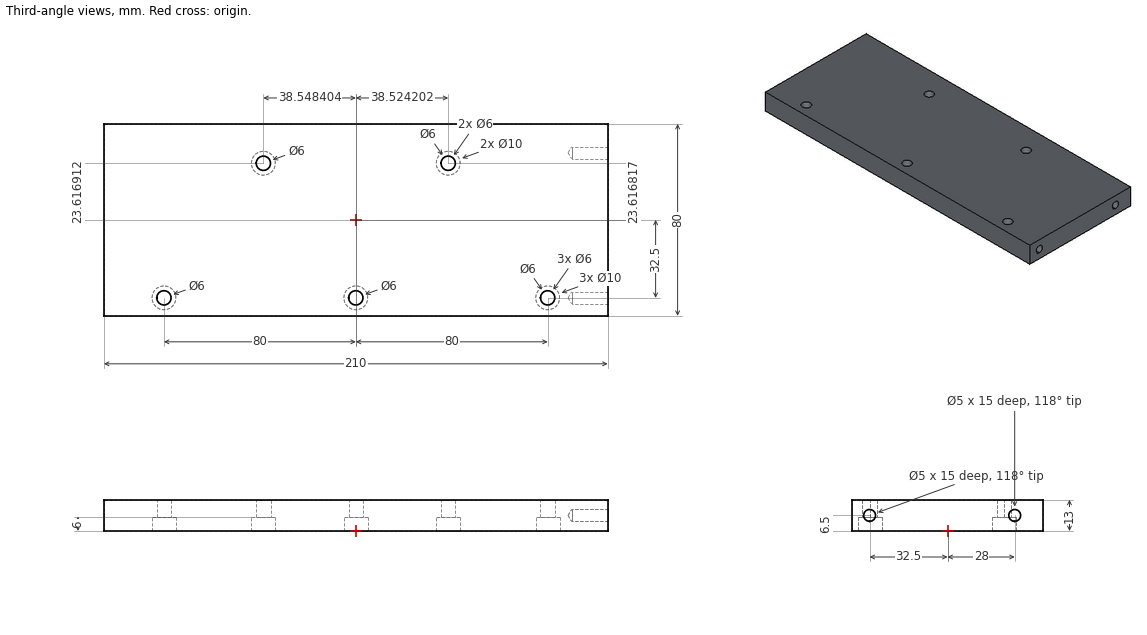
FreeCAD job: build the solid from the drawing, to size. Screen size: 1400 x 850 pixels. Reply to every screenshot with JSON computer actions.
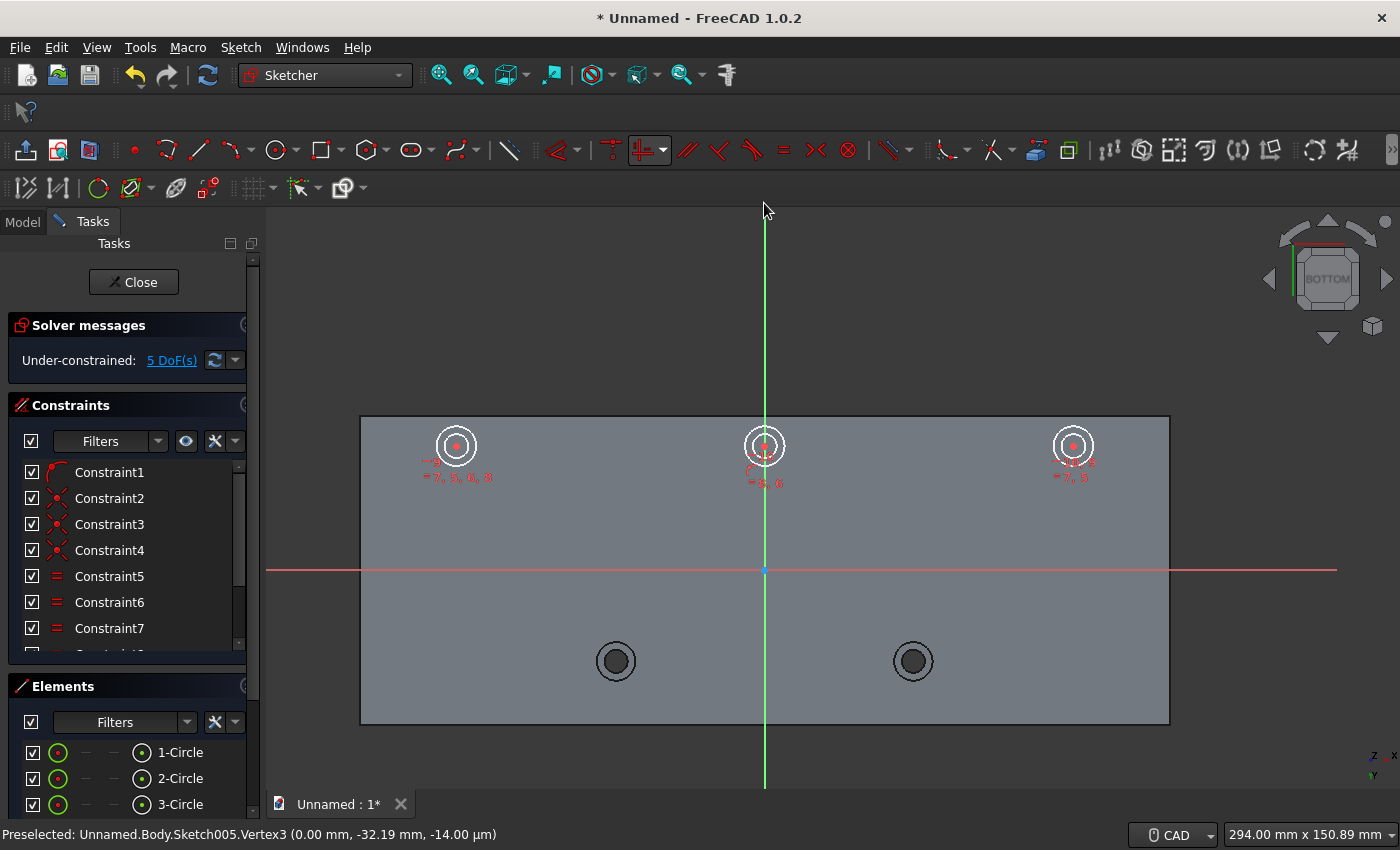
{"action": "key", "text": "d"}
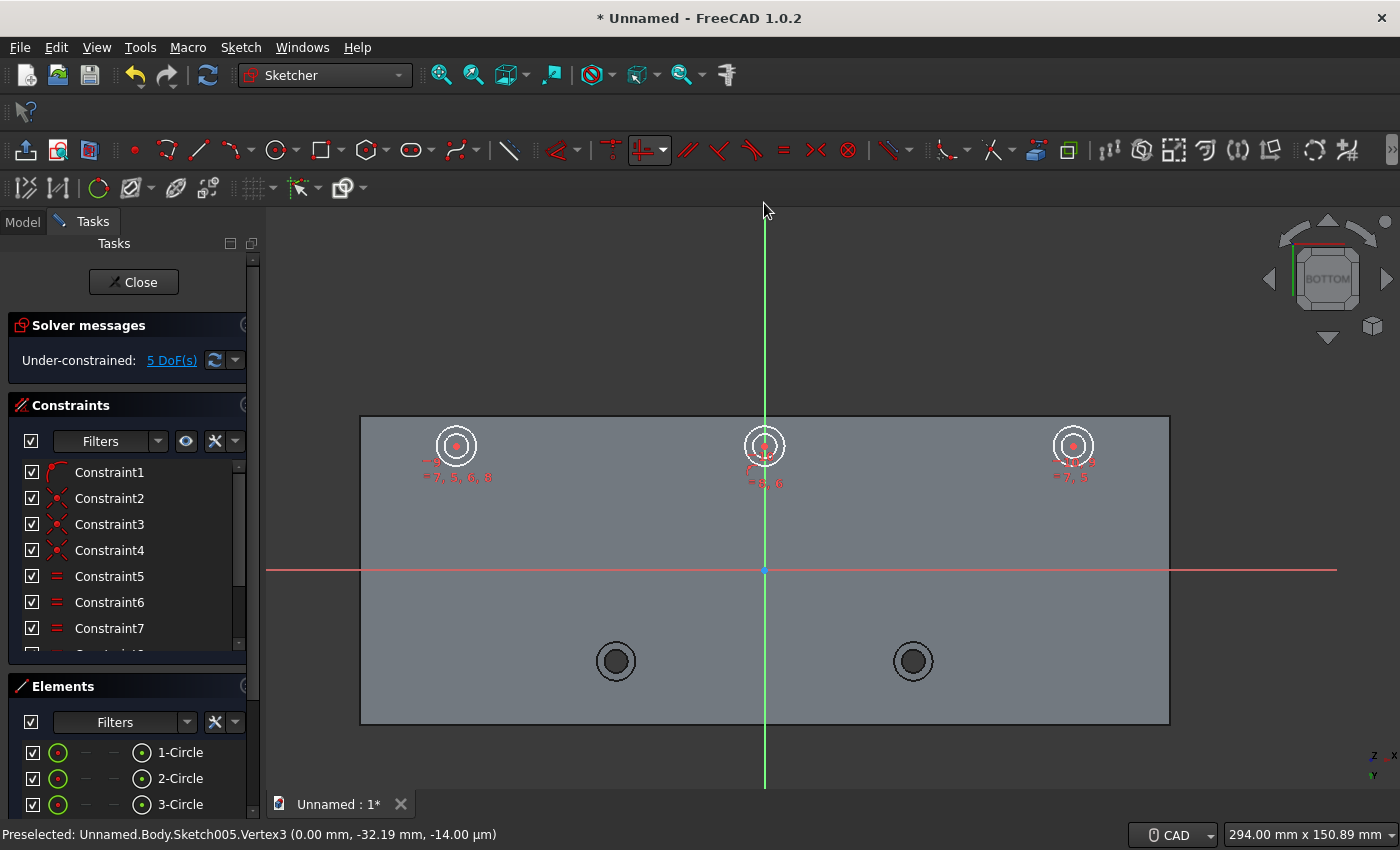
{"action": "scroll", "coordinate": [1059, 432], "scroll_direction": "up", "scroll_amount": 3}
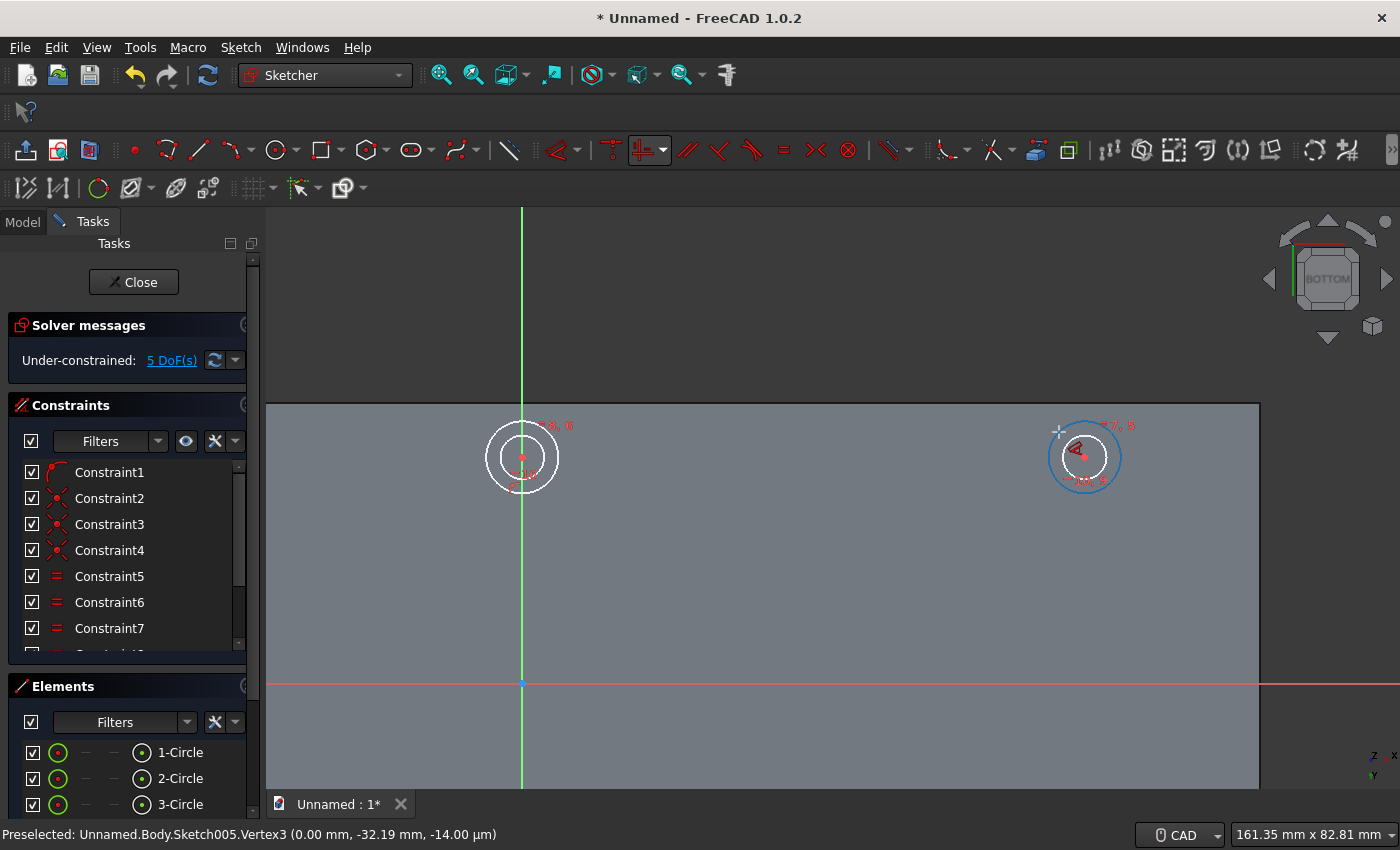
{"action": "left_click", "coordinate": [1059, 432]}
{"action": "left_click", "coordinate": [1036, 410]}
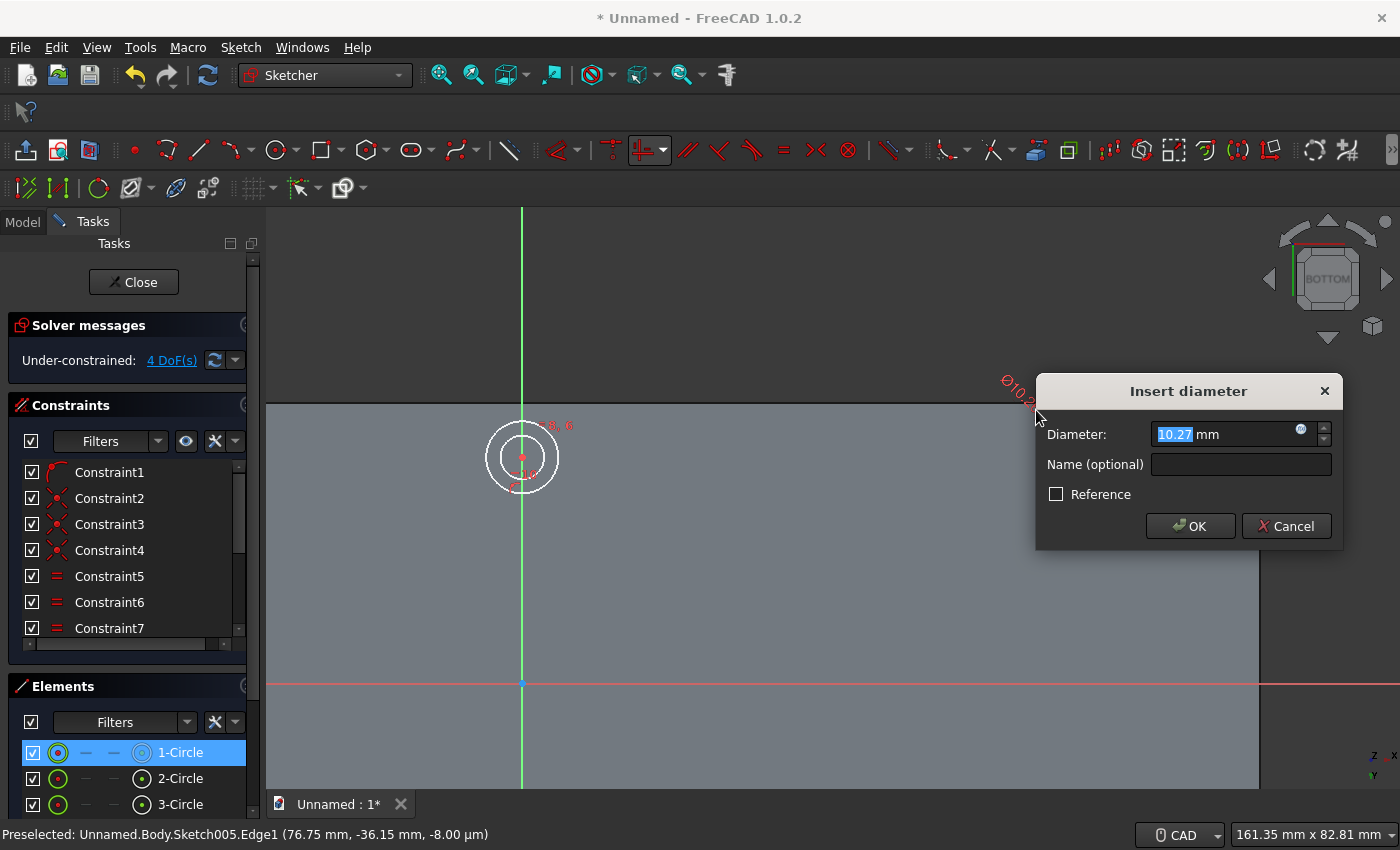
{"action": "type", "text": "10"}
{"action": "key", "text": "Return"}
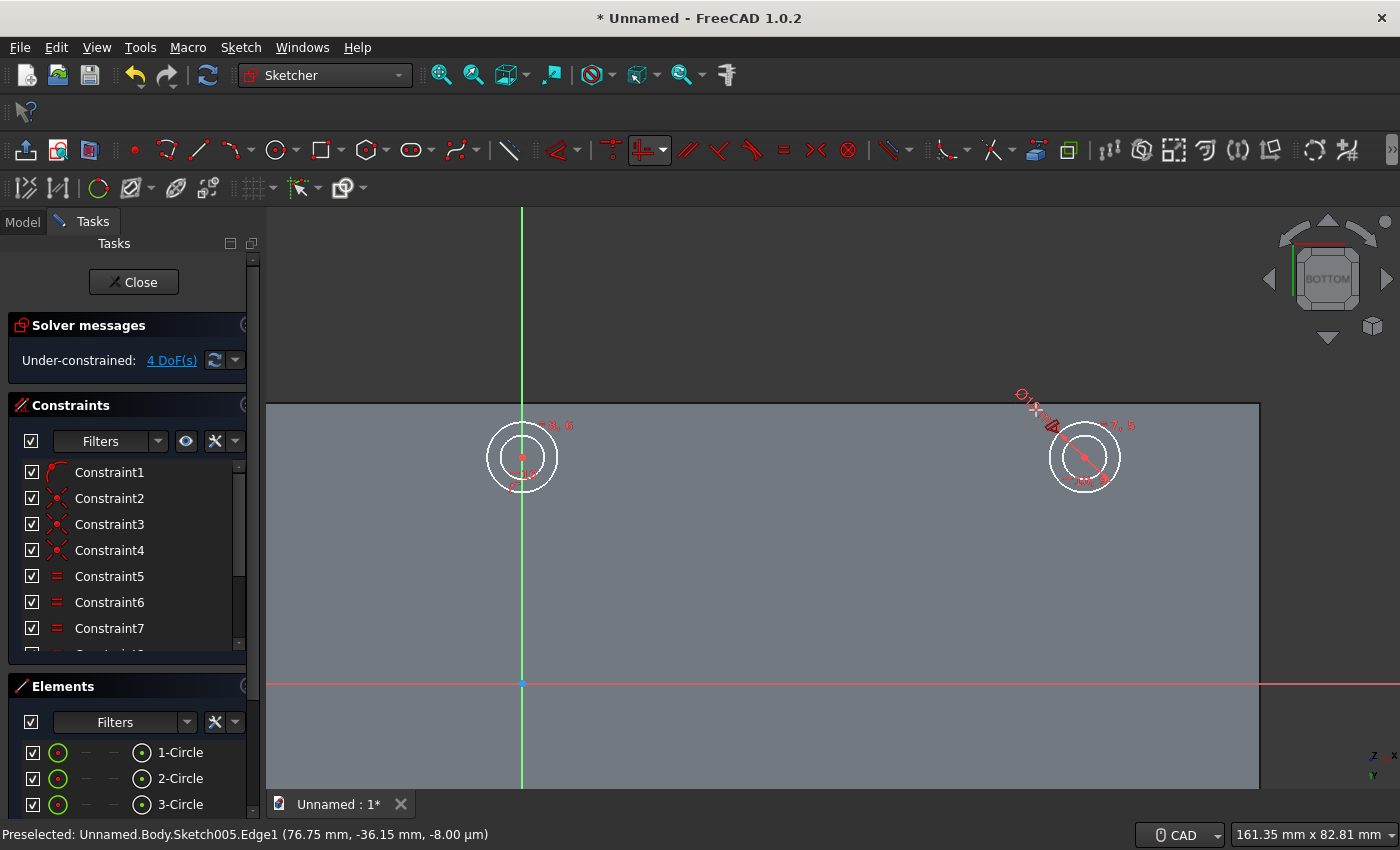
{"action": "left_click", "coordinate": [1100, 442]}
{"action": "left_click", "coordinate": [1123, 419]}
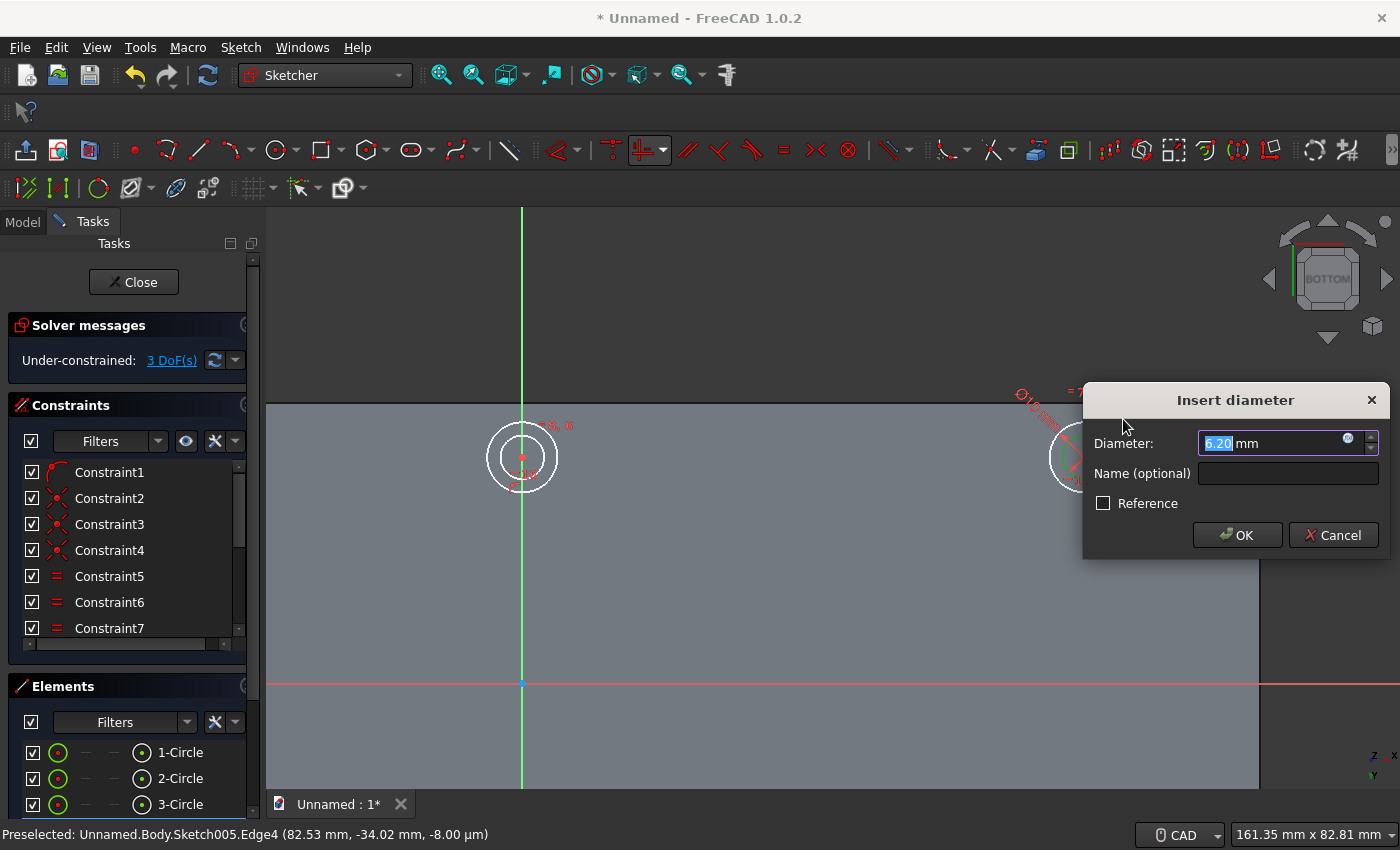
{"action": "type", "text": "6"}
{"action": "key", "text": "Return"}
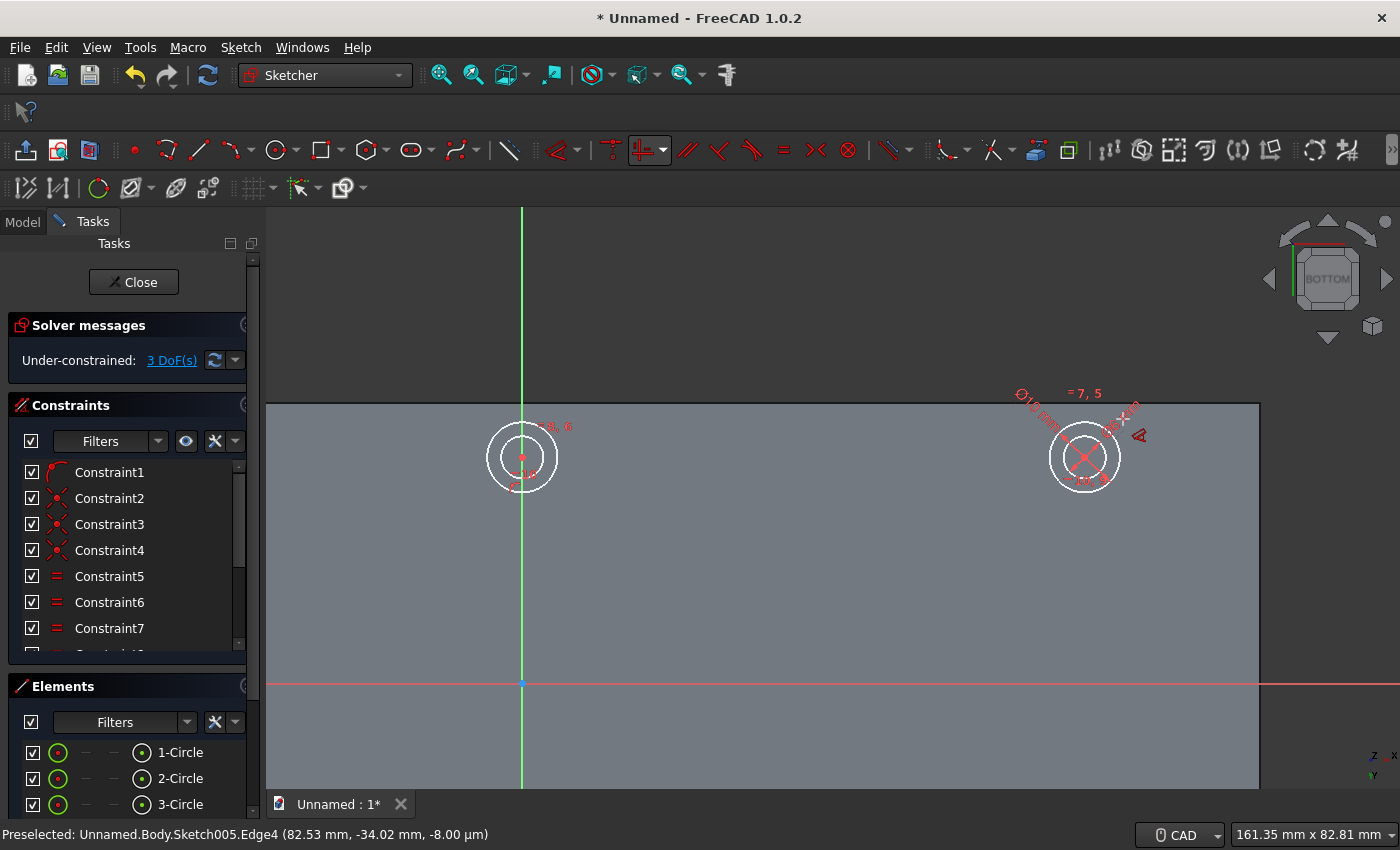
{"action": "left_click", "coordinate": [1085, 457]}
{"action": "left_click", "coordinate": [804, 718]}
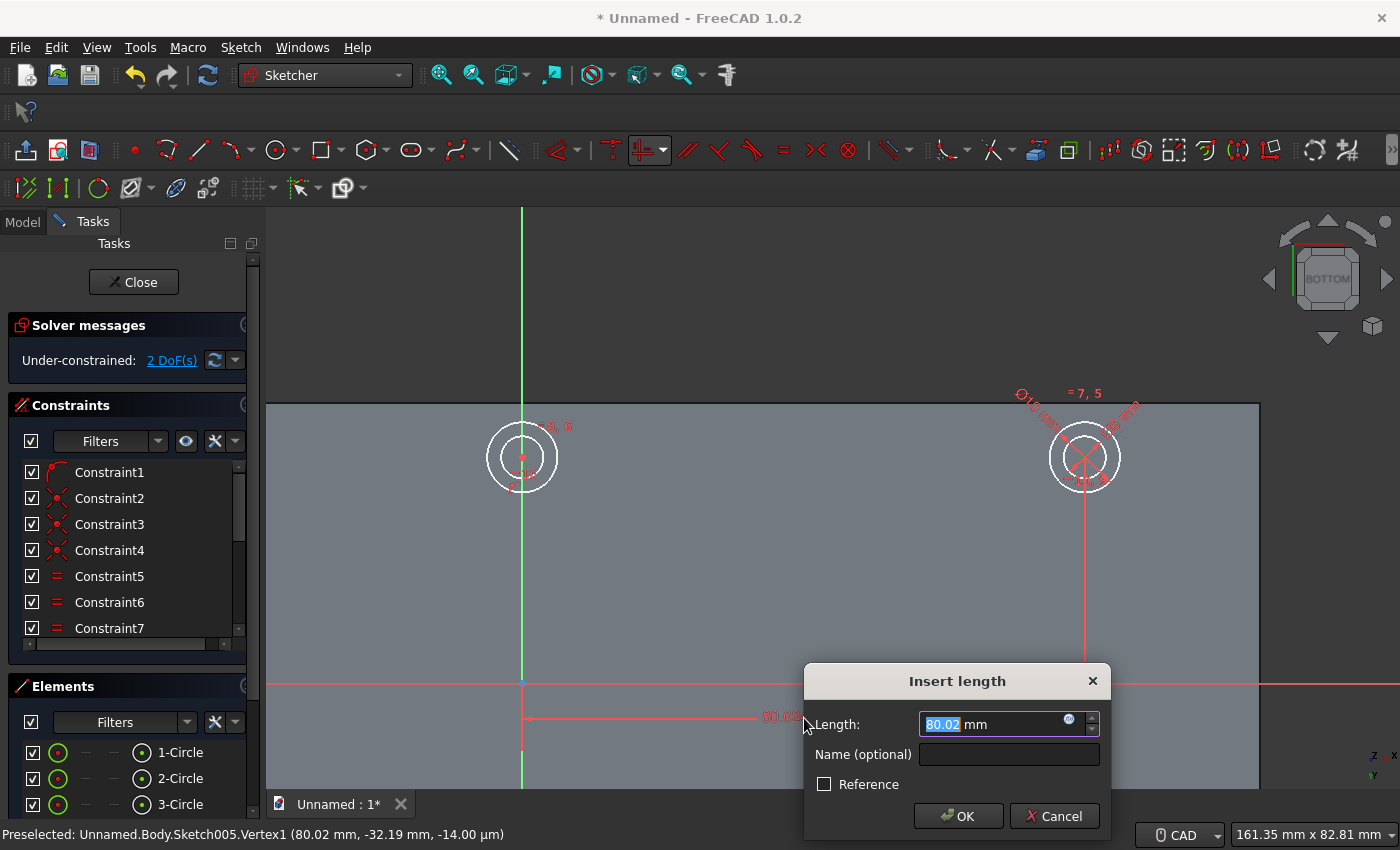
{"action": "type", "text": "80"}
{"action": "key", "text": "Return"}